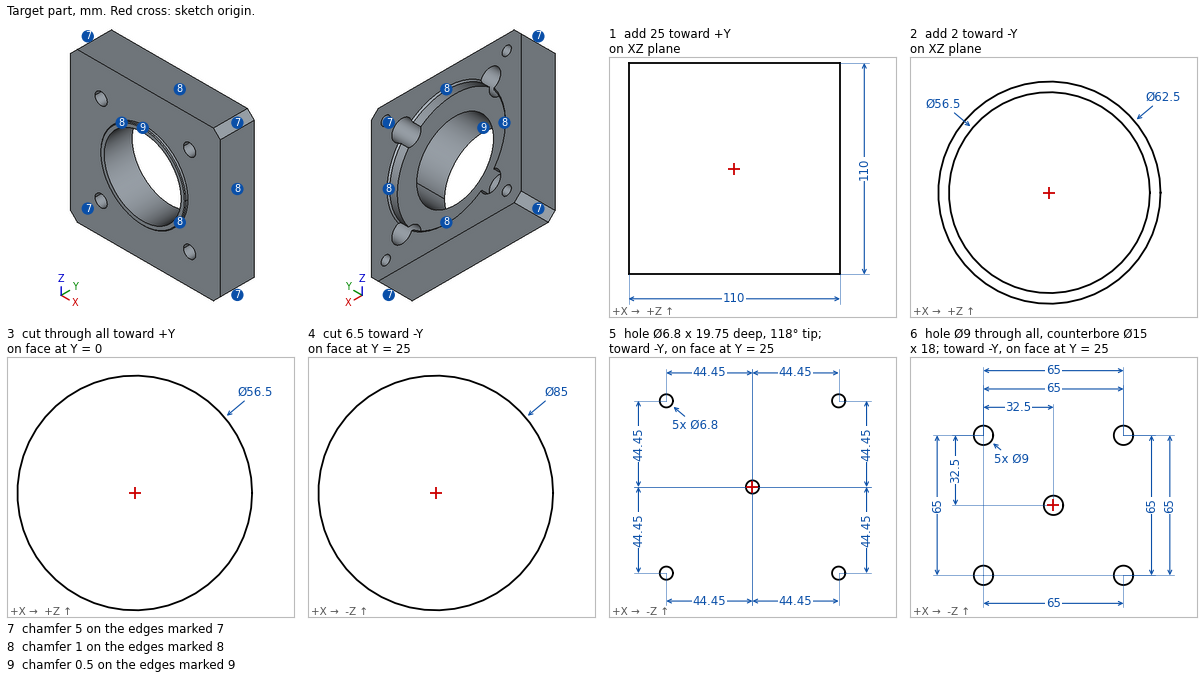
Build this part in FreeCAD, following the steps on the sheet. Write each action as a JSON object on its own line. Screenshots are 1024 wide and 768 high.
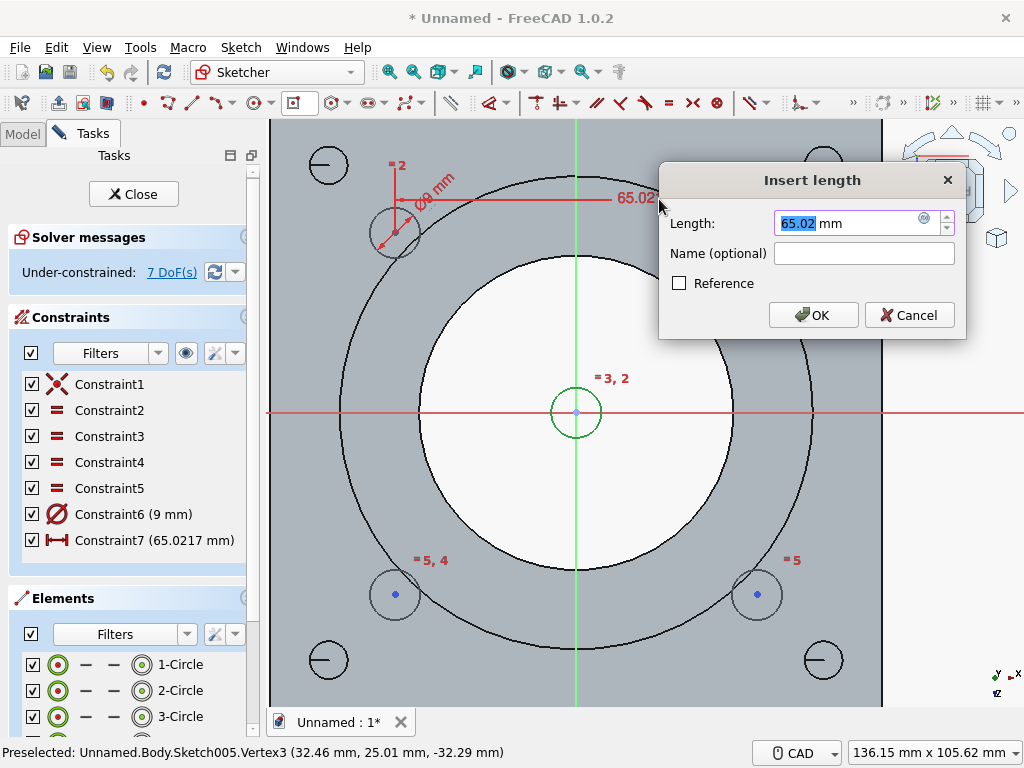
{"action": "type", "text": "65"}
{"action": "key", "text": "Return"}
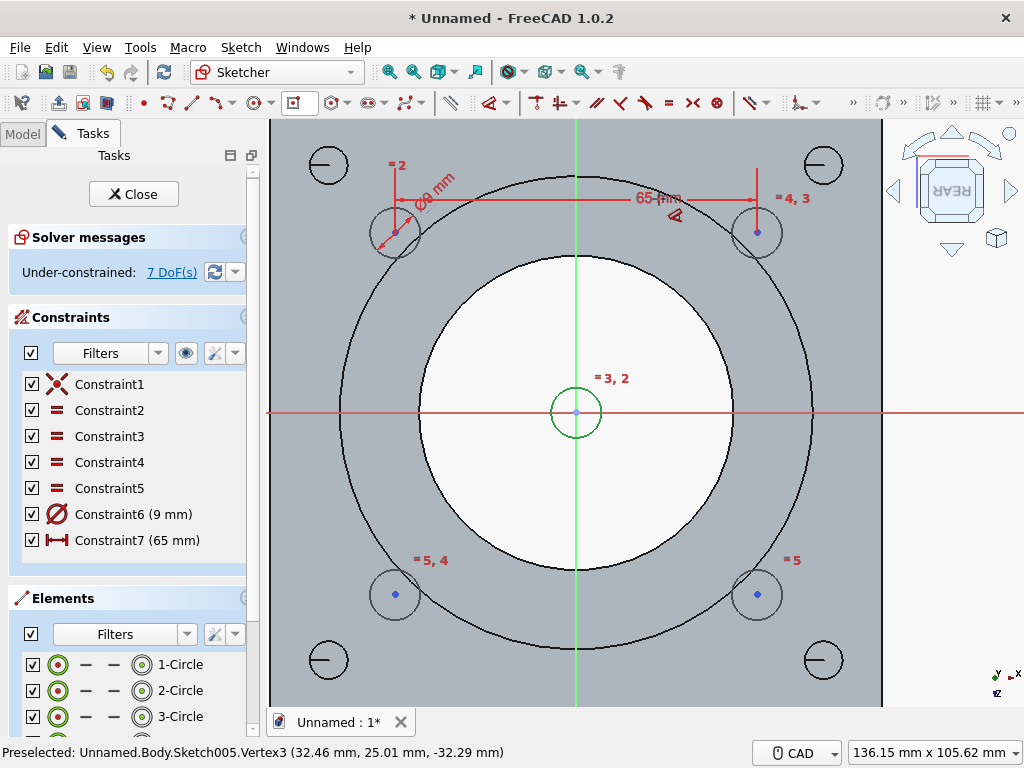
{"action": "left_click", "coordinate": [757, 233]}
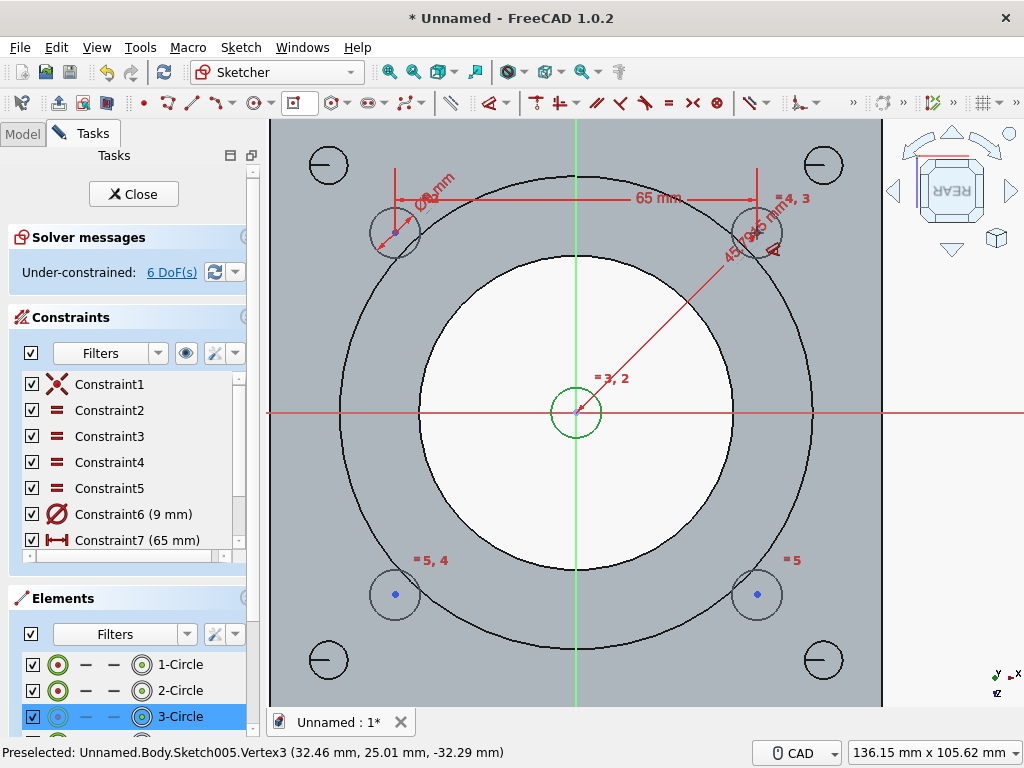
{"action": "left_click", "coordinate": [395, 595]}
{"action": "left_click", "coordinate": [493, 629]}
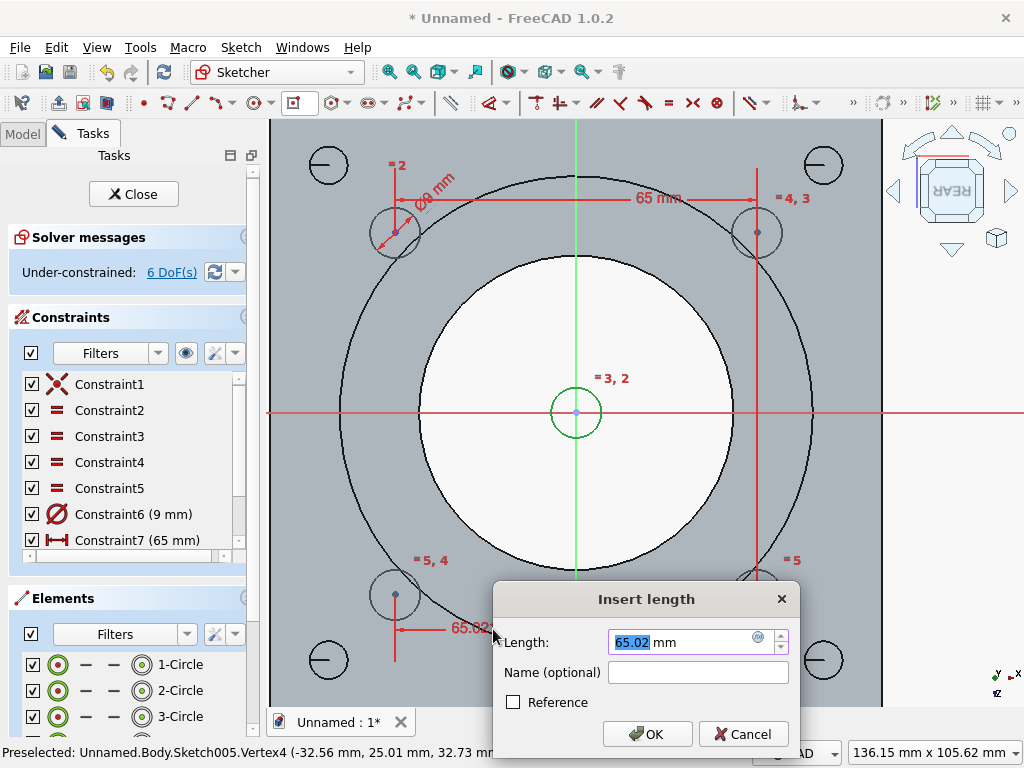
{"action": "type", "text": "65"}
{"action": "key", "text": "Return"}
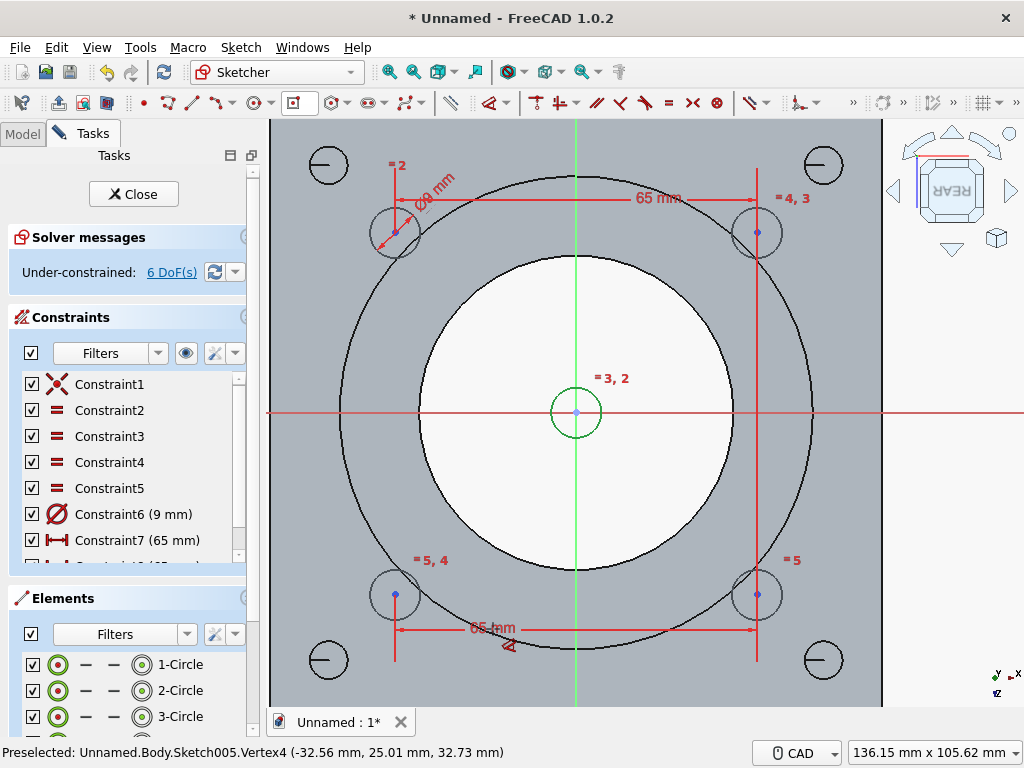
{"action": "left_click", "coordinate": [395, 233]}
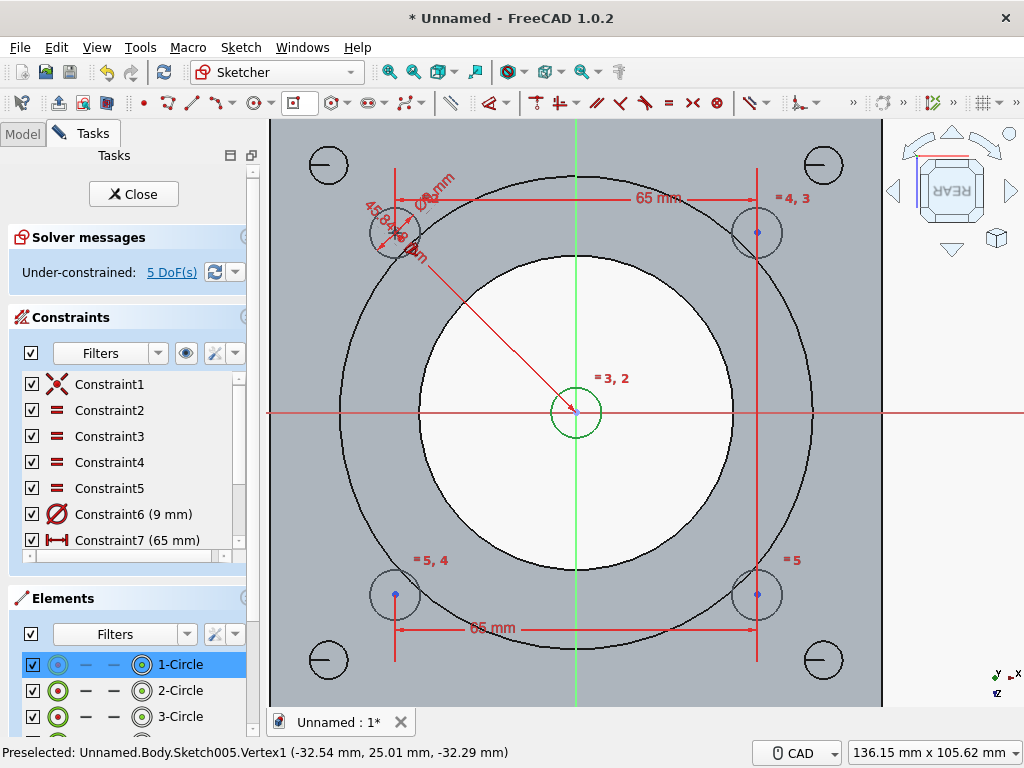
{"action": "left_click", "coordinate": [395, 595]}
{"action": "left_click", "coordinate": [361, 331]}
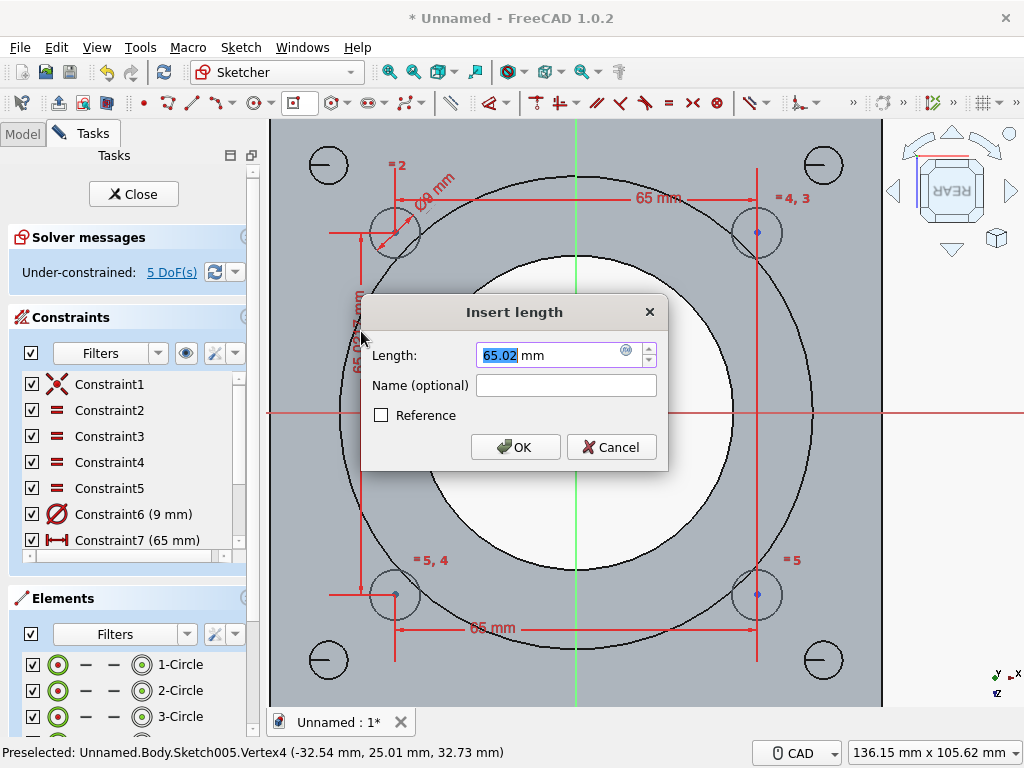
{"action": "type", "text": "65"}
{"action": "key", "text": "Return"}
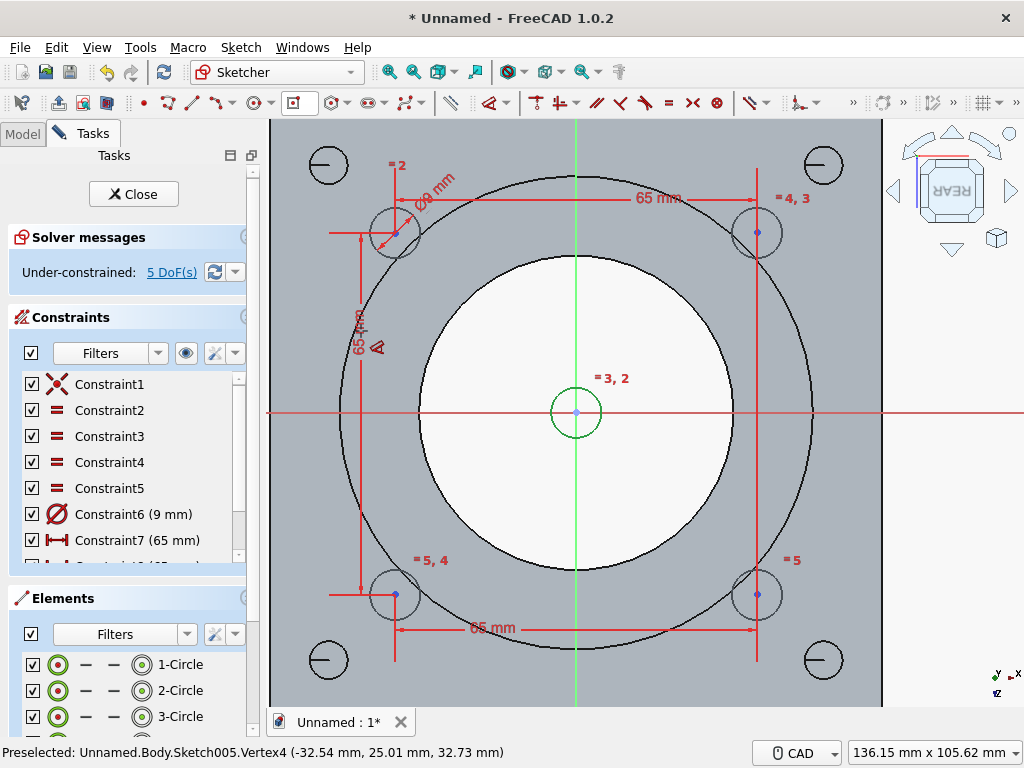
{"action": "left_click", "coordinate": [757, 233]}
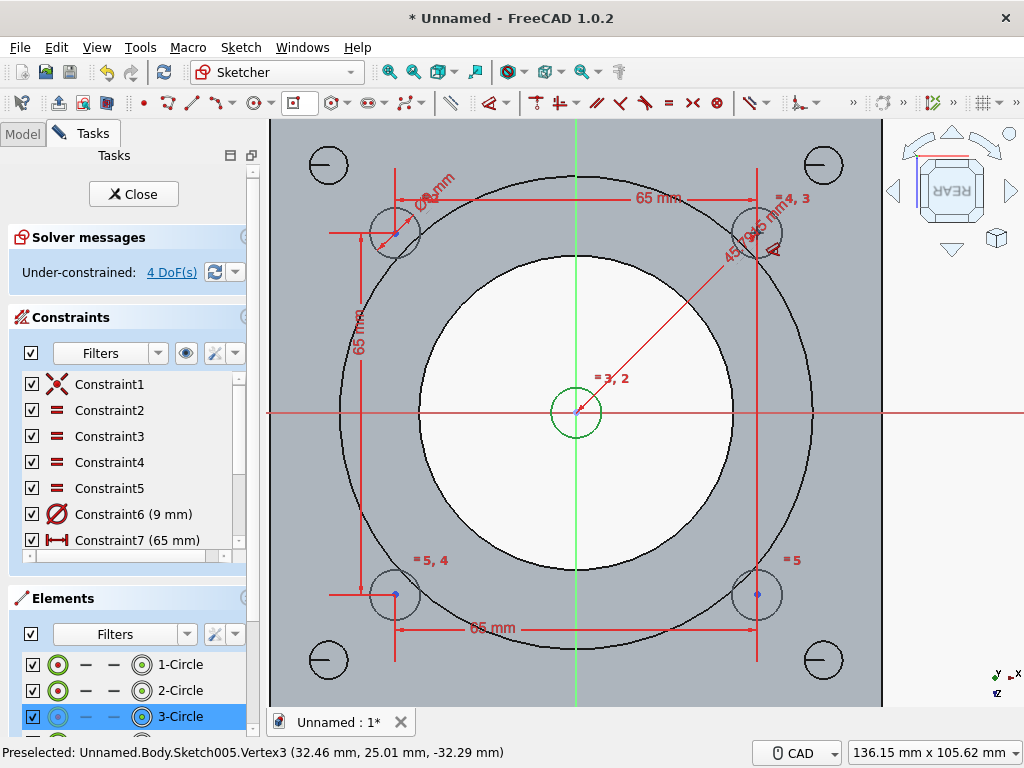
{"action": "left_click", "coordinate": [395, 595]}
{"action": "left_click", "coordinate": [361, 497]}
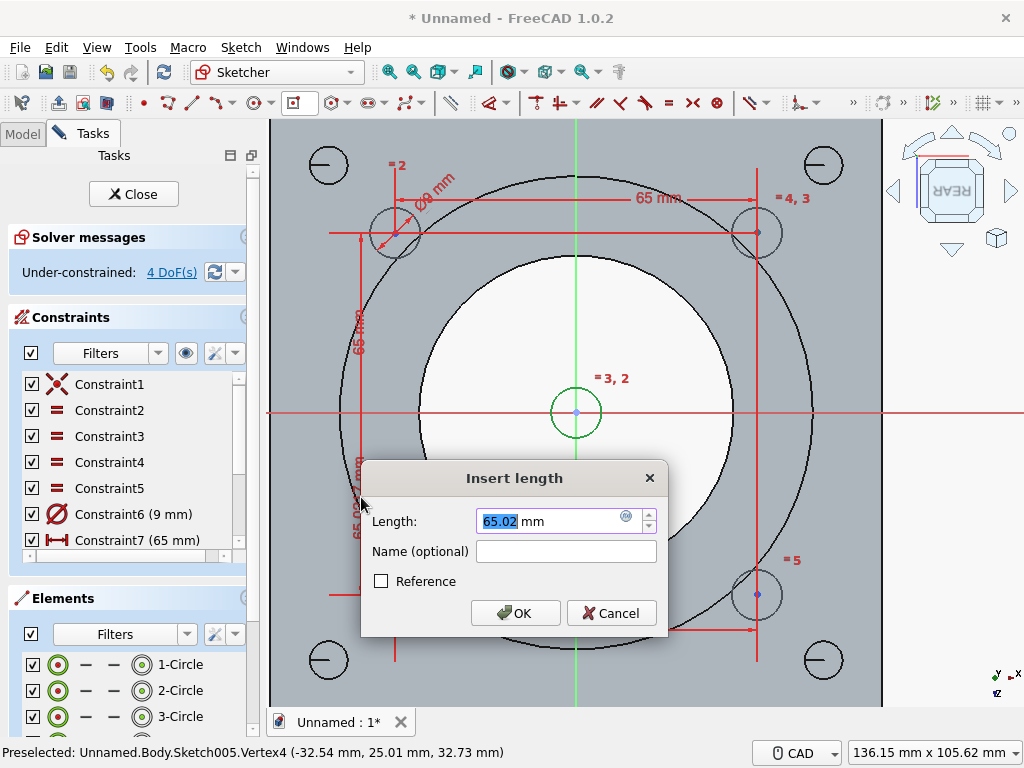
{"action": "type", "text": "65"}
{"action": "key", "text": "Return"}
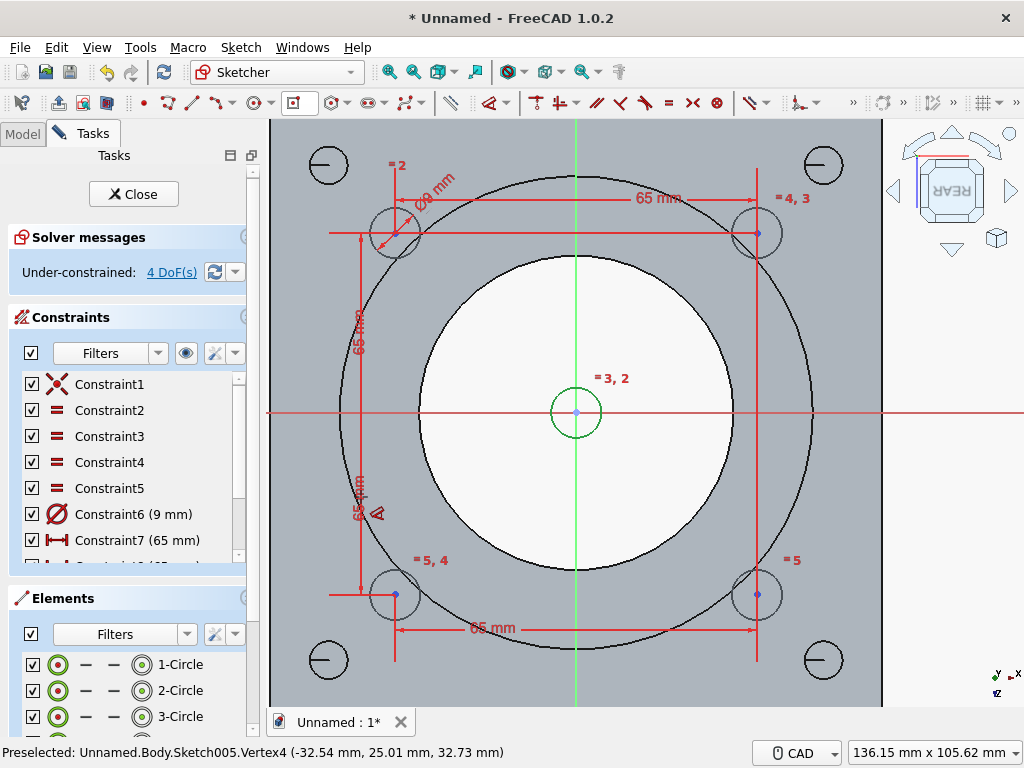
{"action": "left_click", "coordinate": [395, 595]}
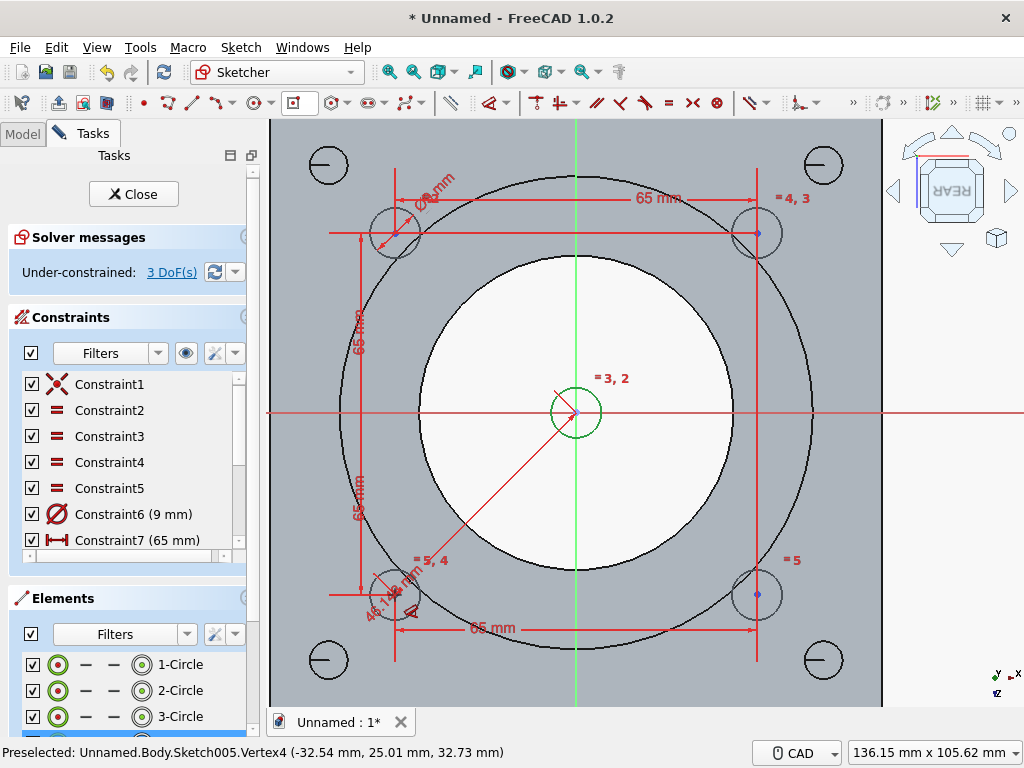
{"action": "left_click", "coordinate": [757, 595]}
{"action": "left_click", "coordinate": [659, 629]}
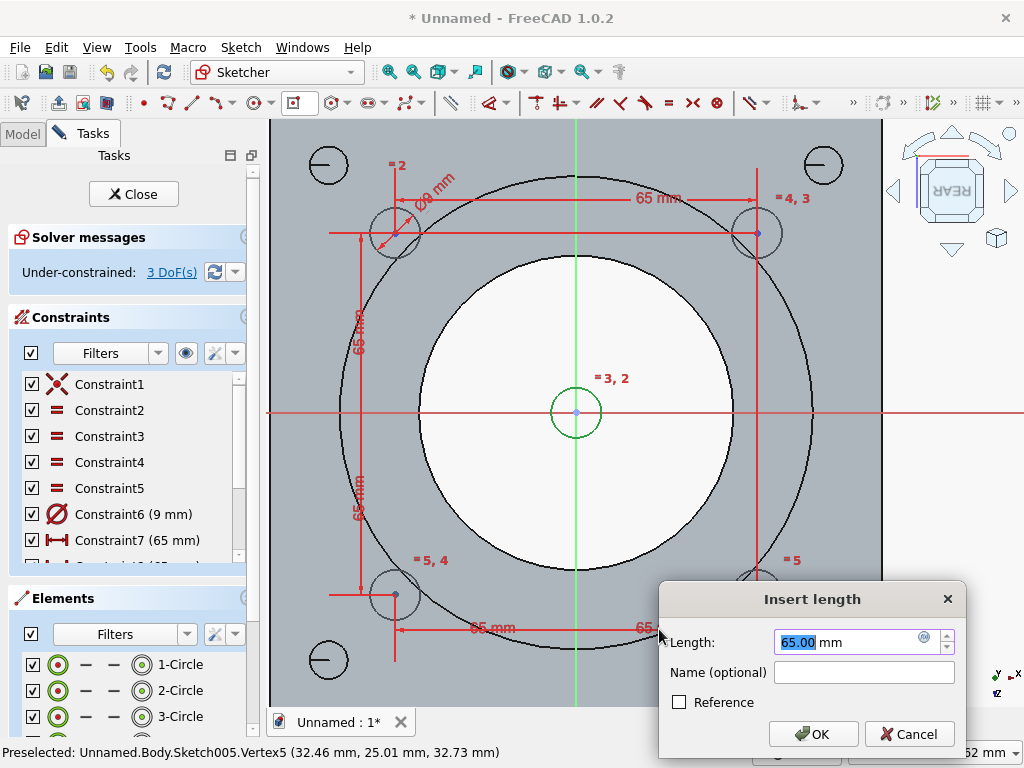
{"action": "type", "text": "65"}
{"action": "key", "text": "Return"}